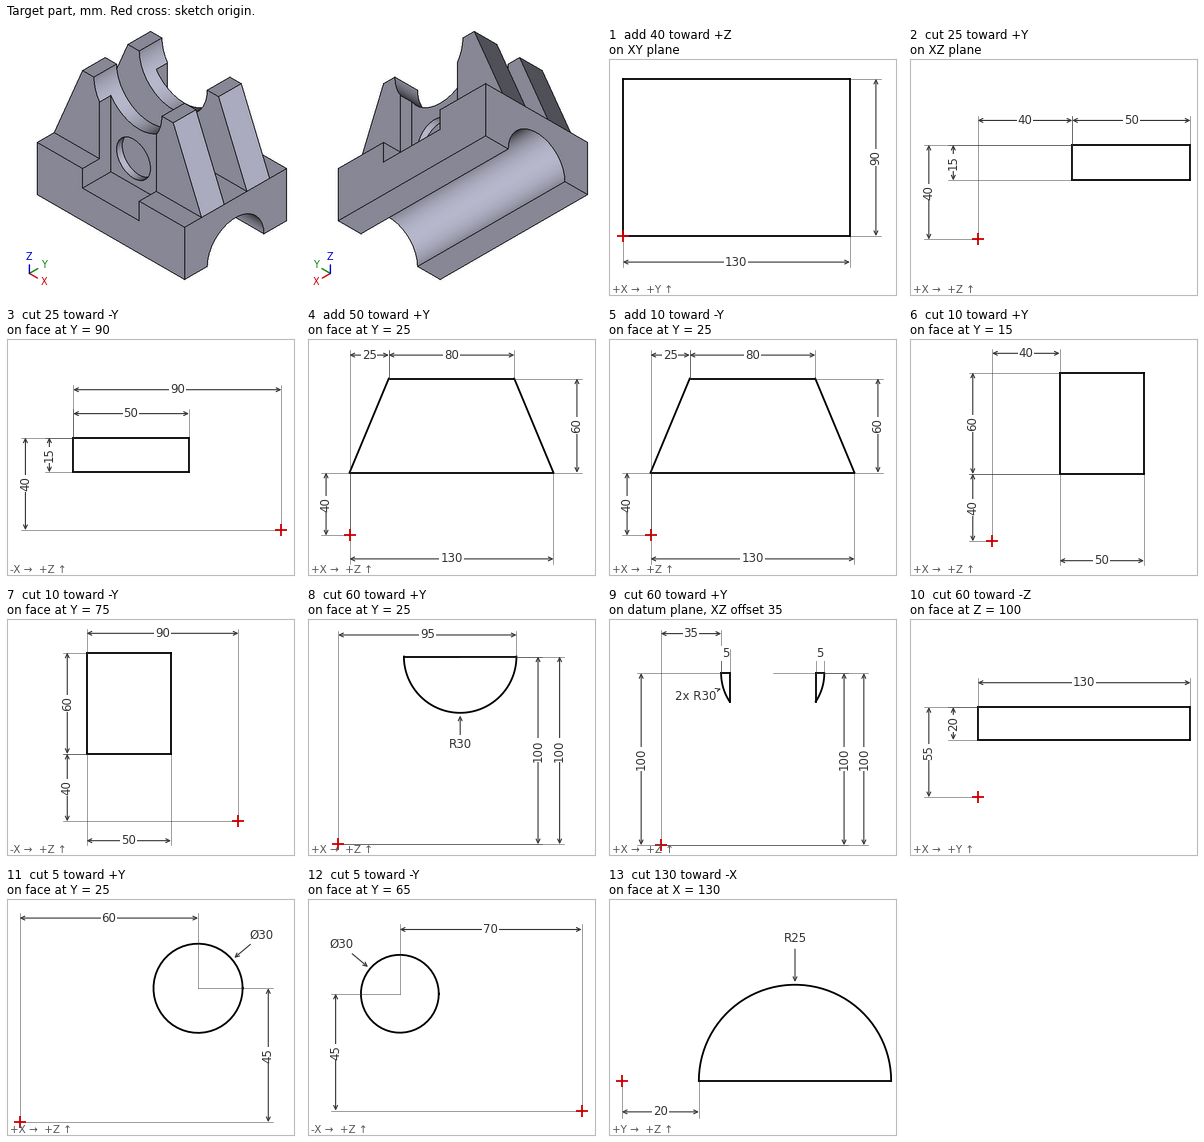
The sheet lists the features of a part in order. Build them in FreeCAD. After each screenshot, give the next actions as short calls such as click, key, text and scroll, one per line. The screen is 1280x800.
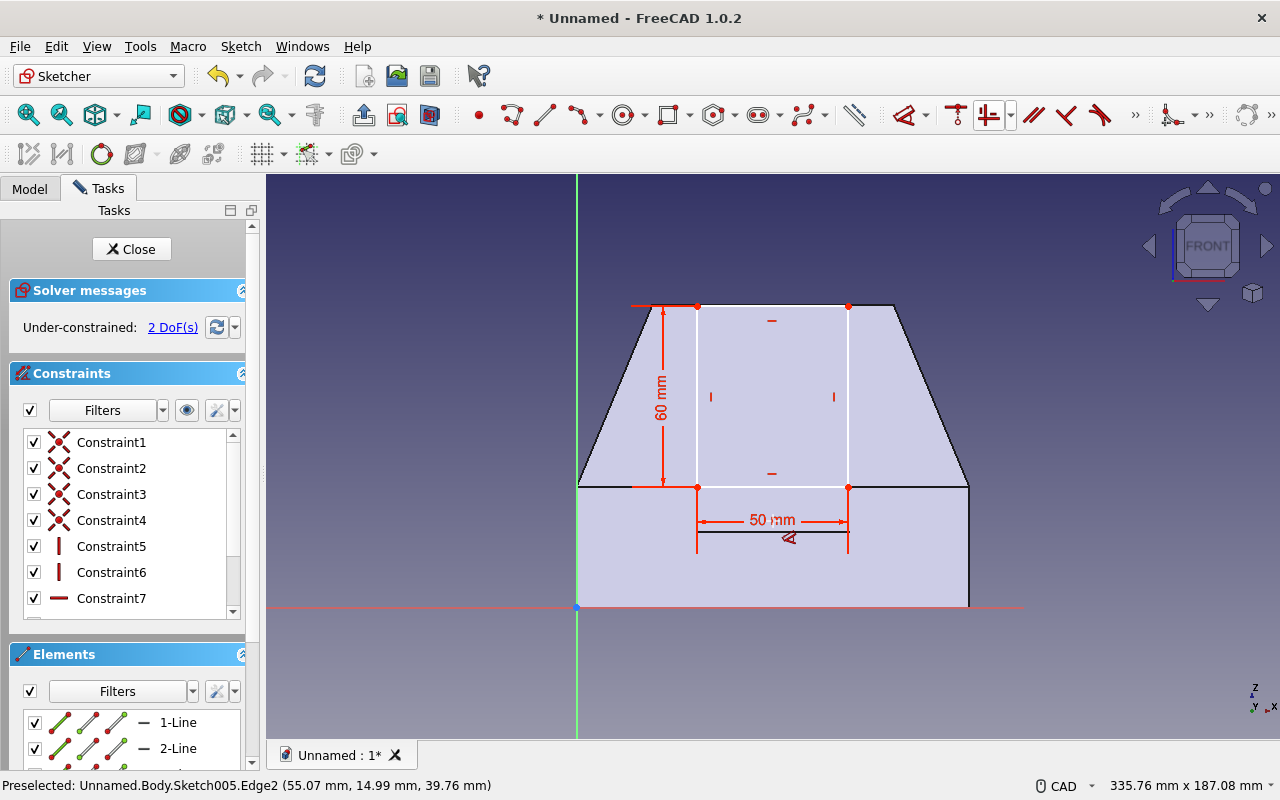
click(697, 306)
click(637, 642)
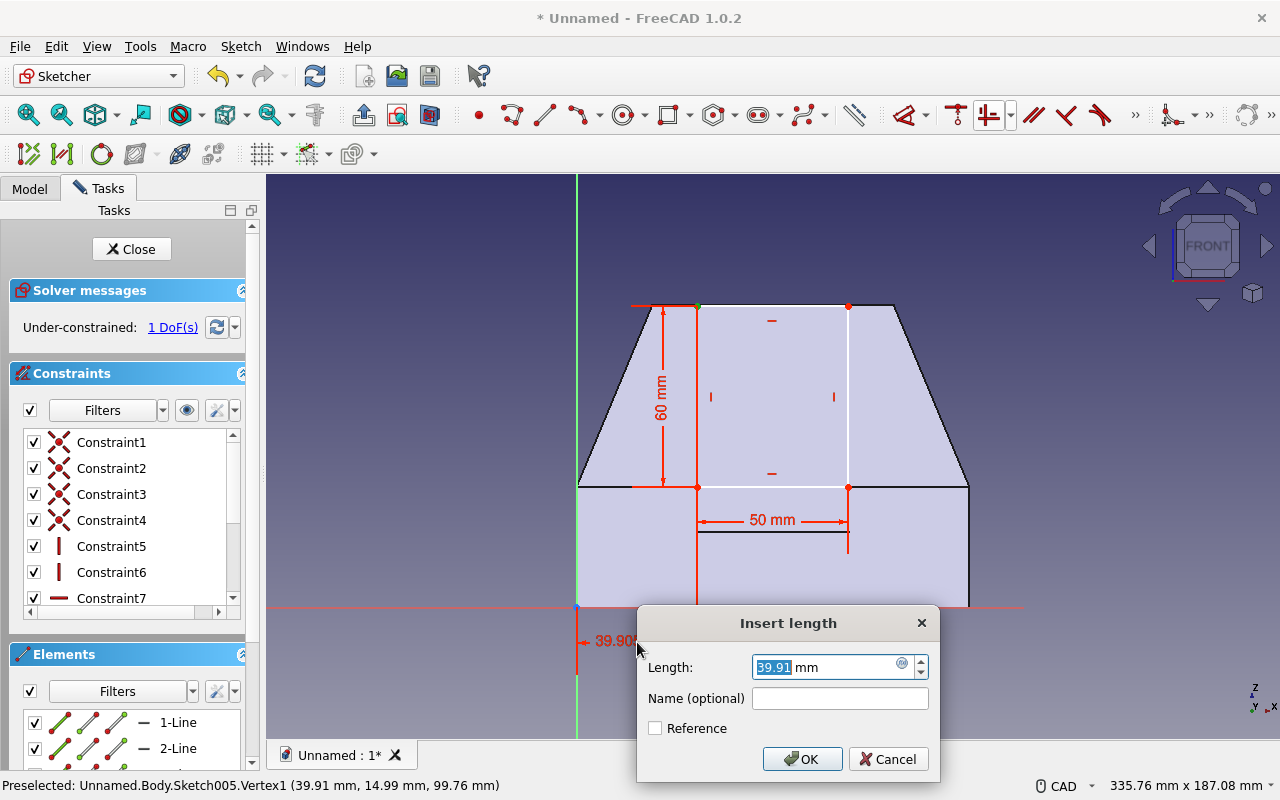
text(40)
key(Return)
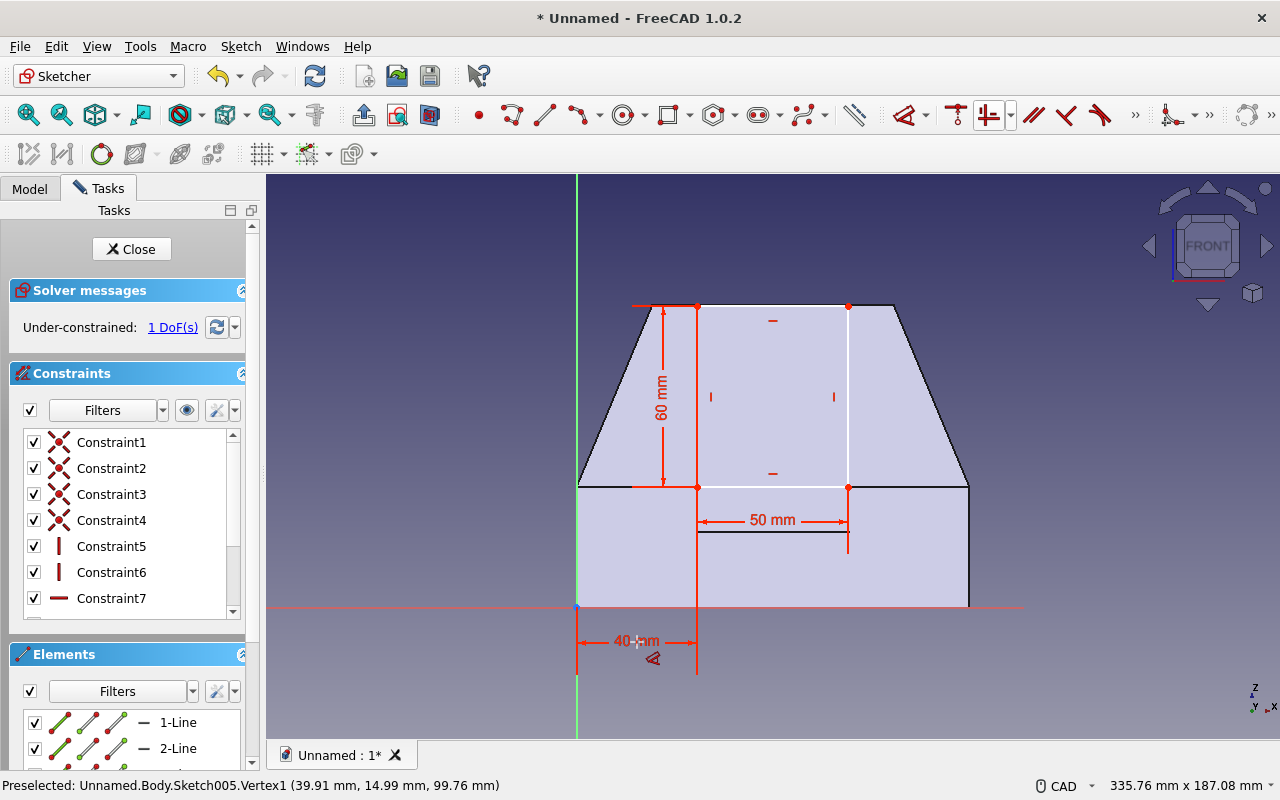
click(697, 487)
click(543, 547)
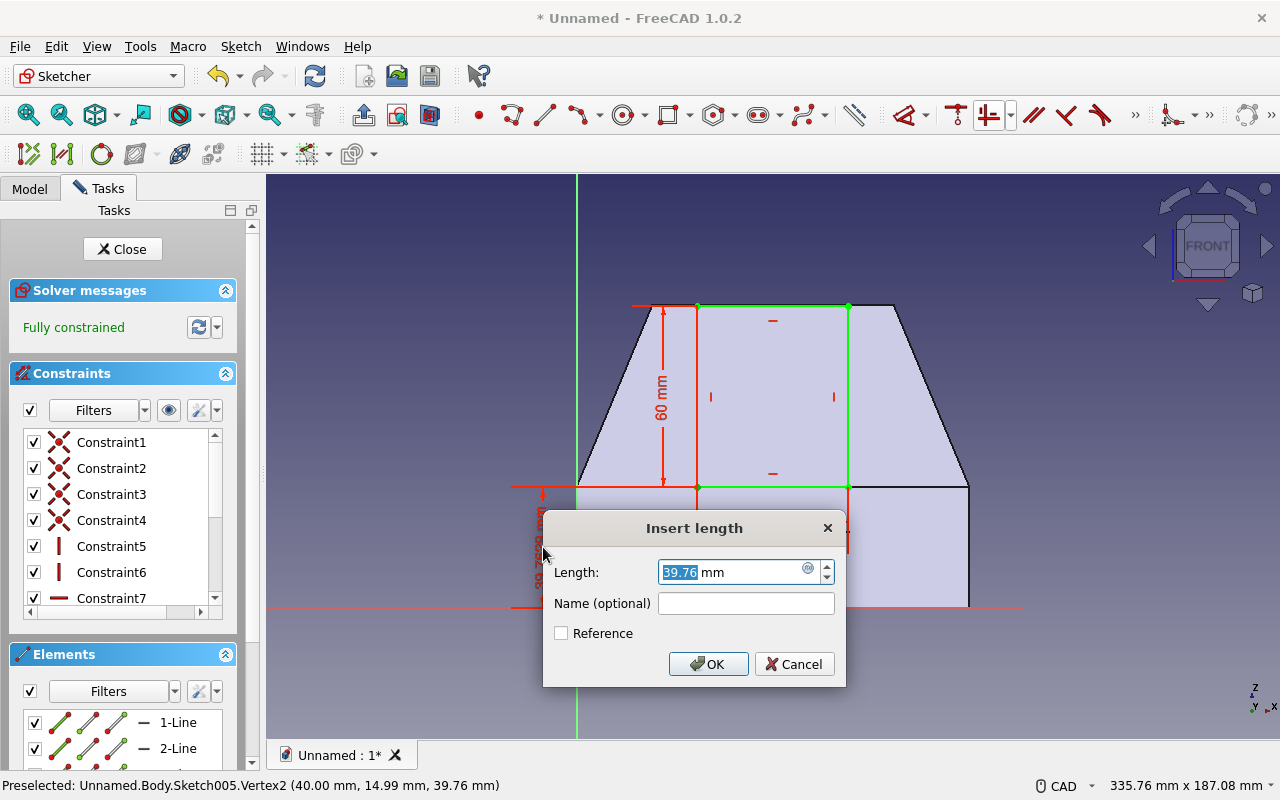
text(40)
key(Return)
key(Escape)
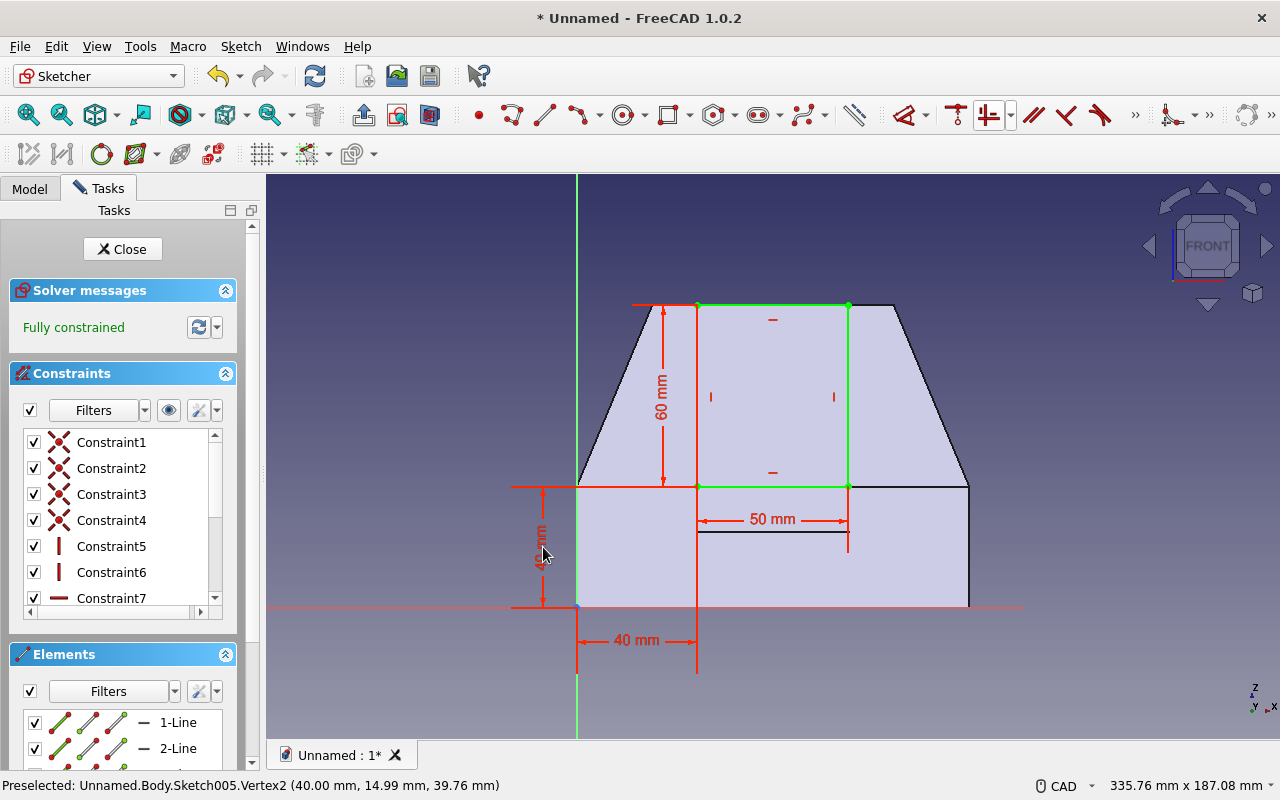
click(123, 249)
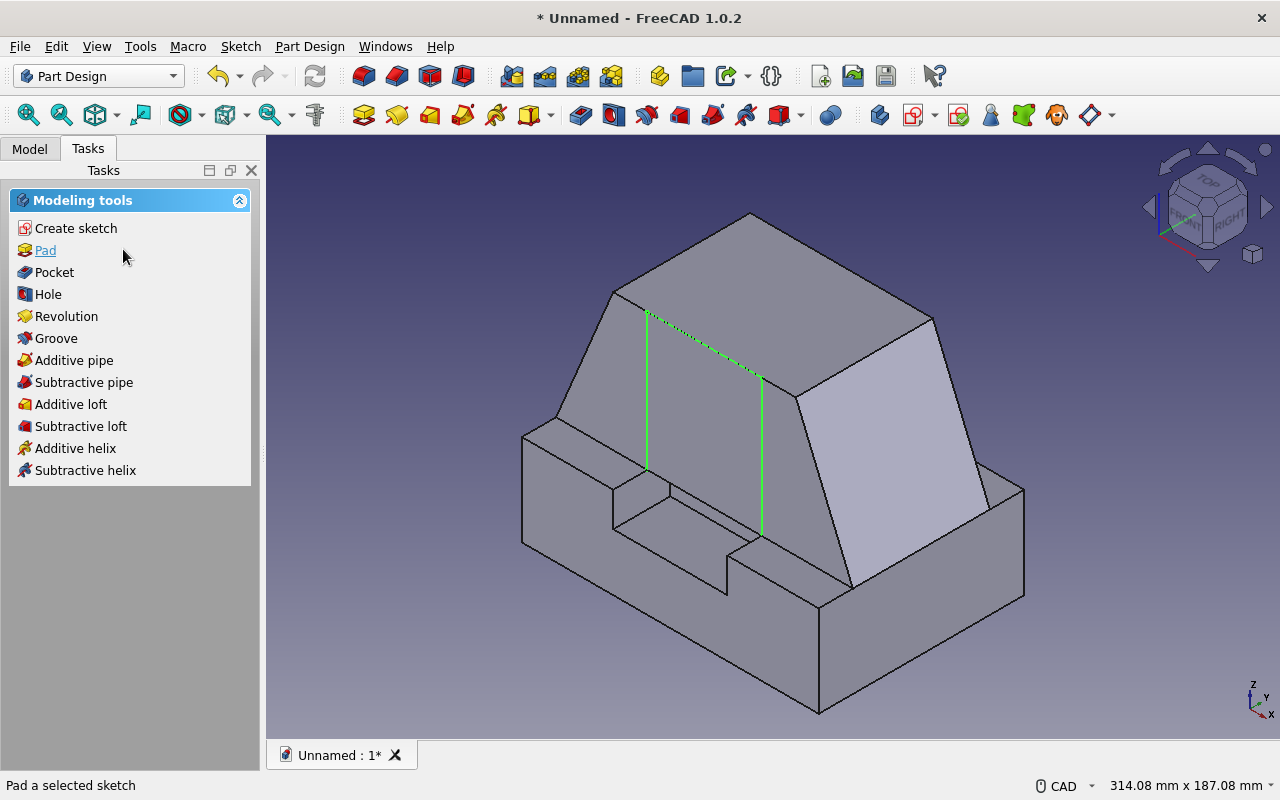
click(581, 116)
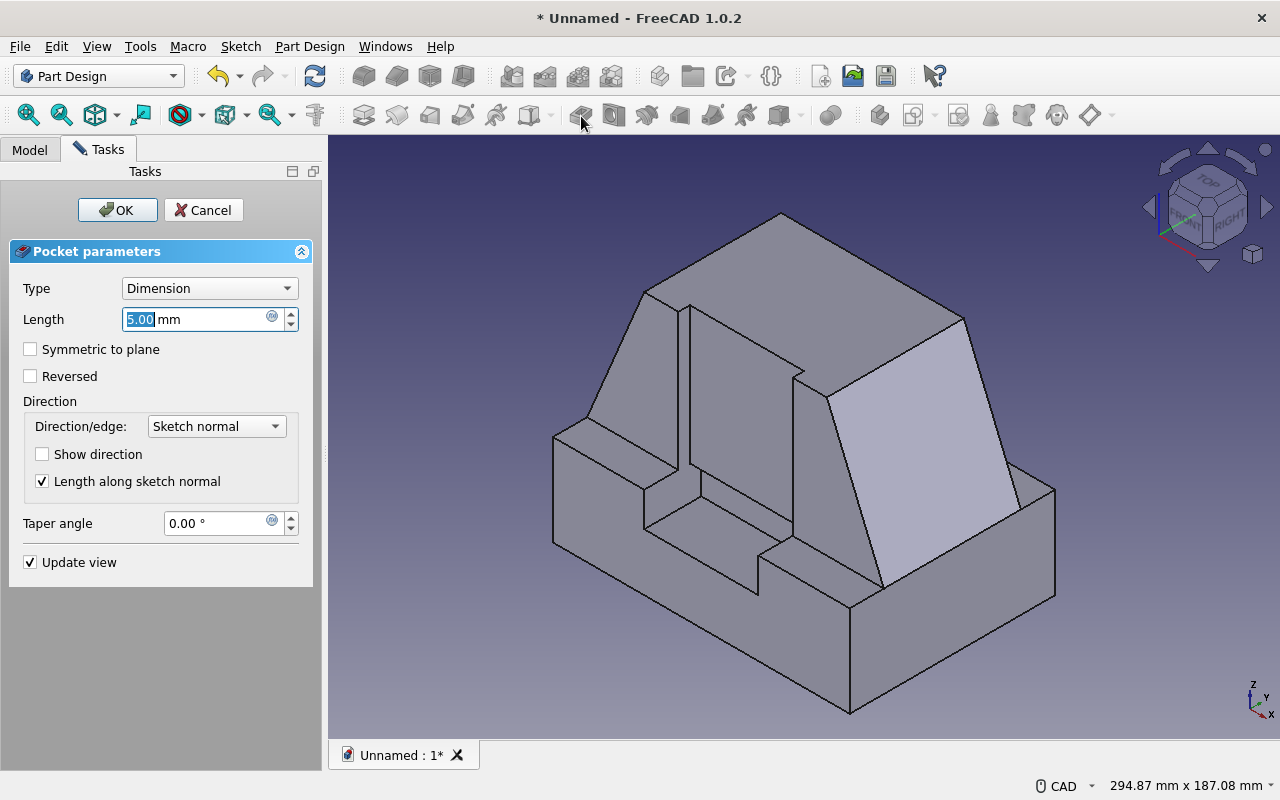
text(10)
key(Tab)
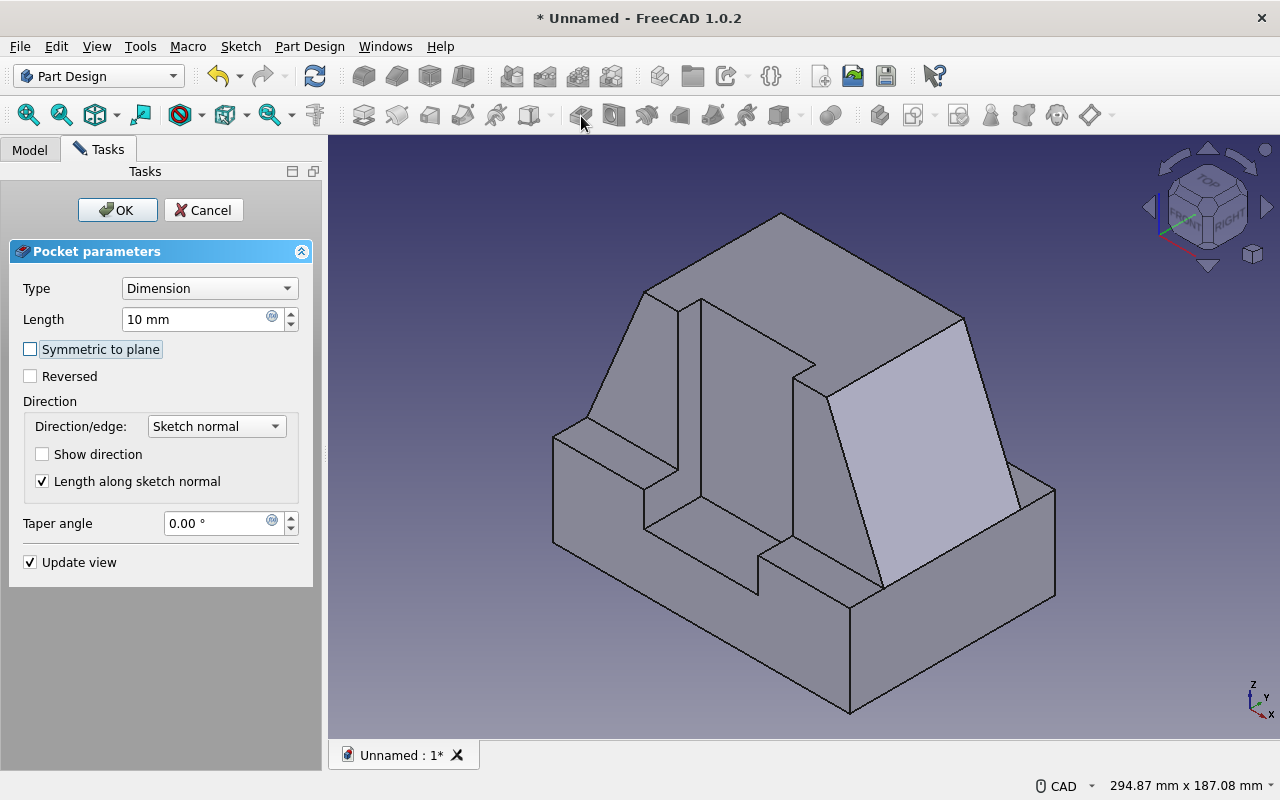
click(118, 210)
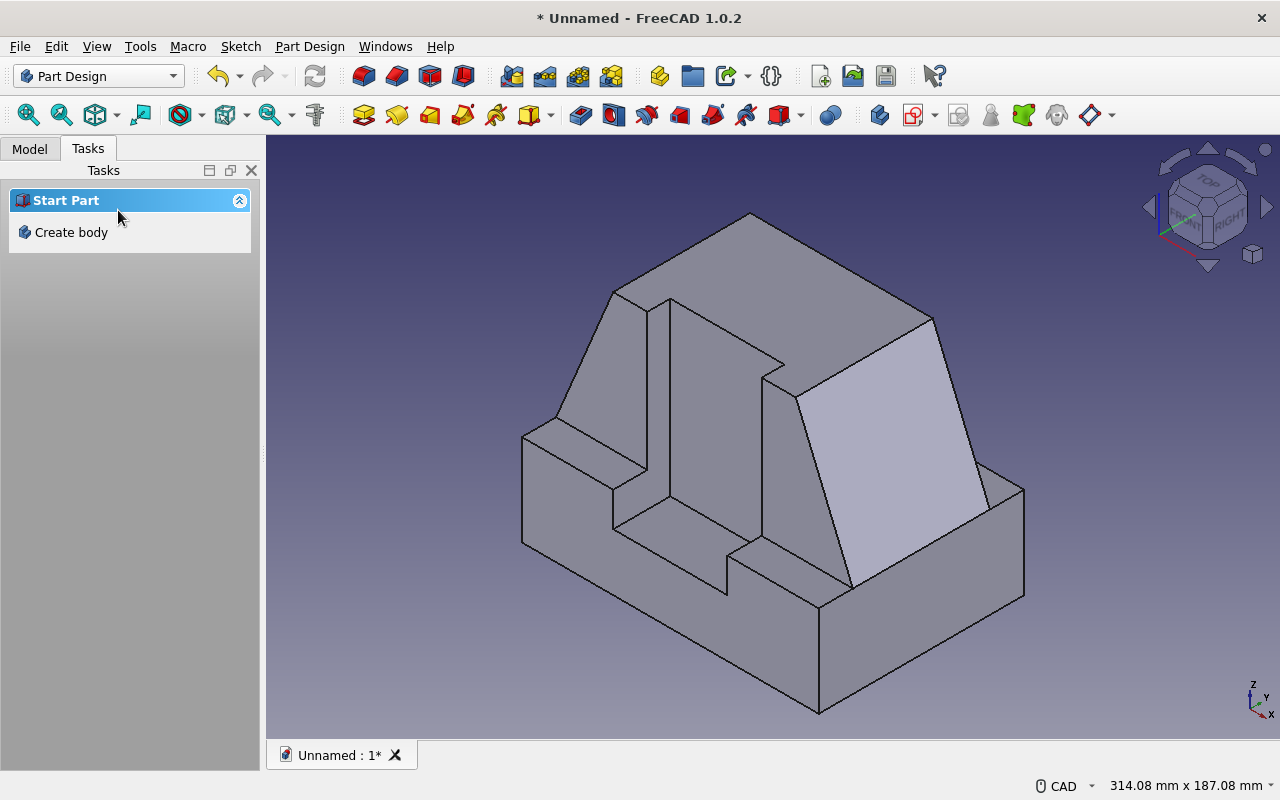
key(4)